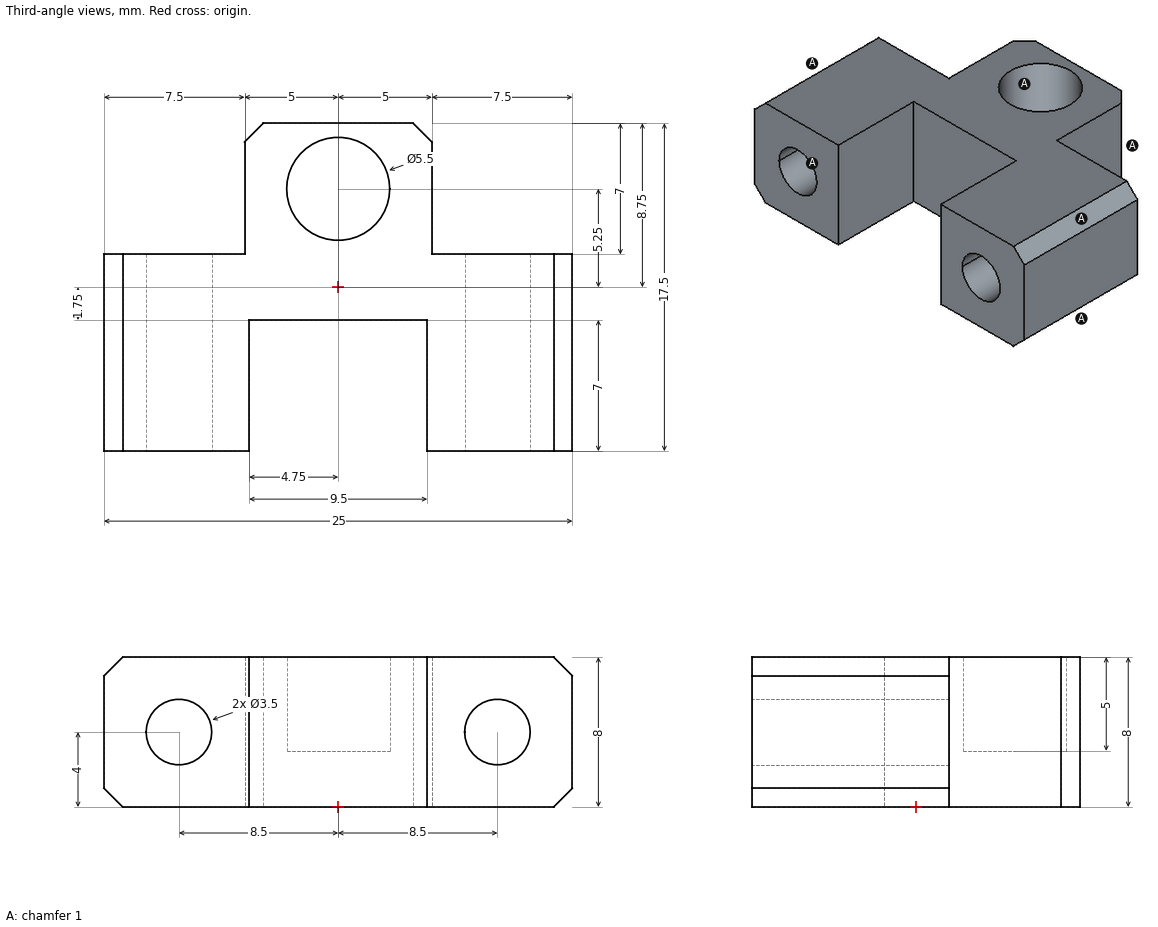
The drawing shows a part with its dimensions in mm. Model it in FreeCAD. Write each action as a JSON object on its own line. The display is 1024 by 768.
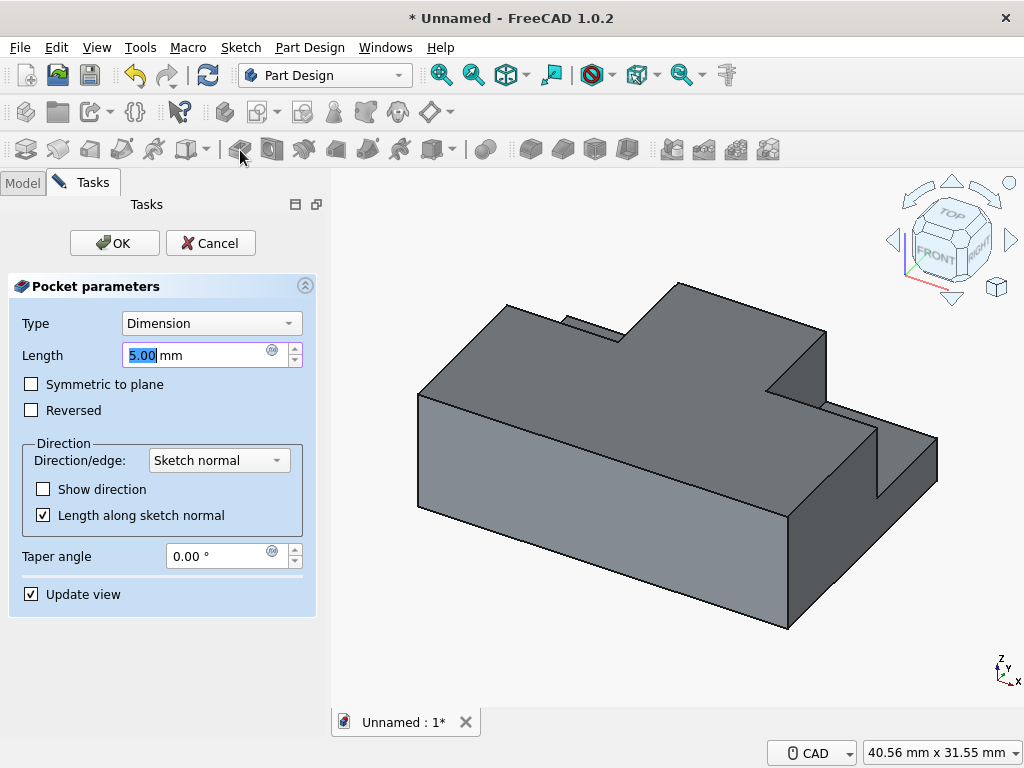
{"action": "type", "text": "8"}
{"action": "key", "text": "Tab"}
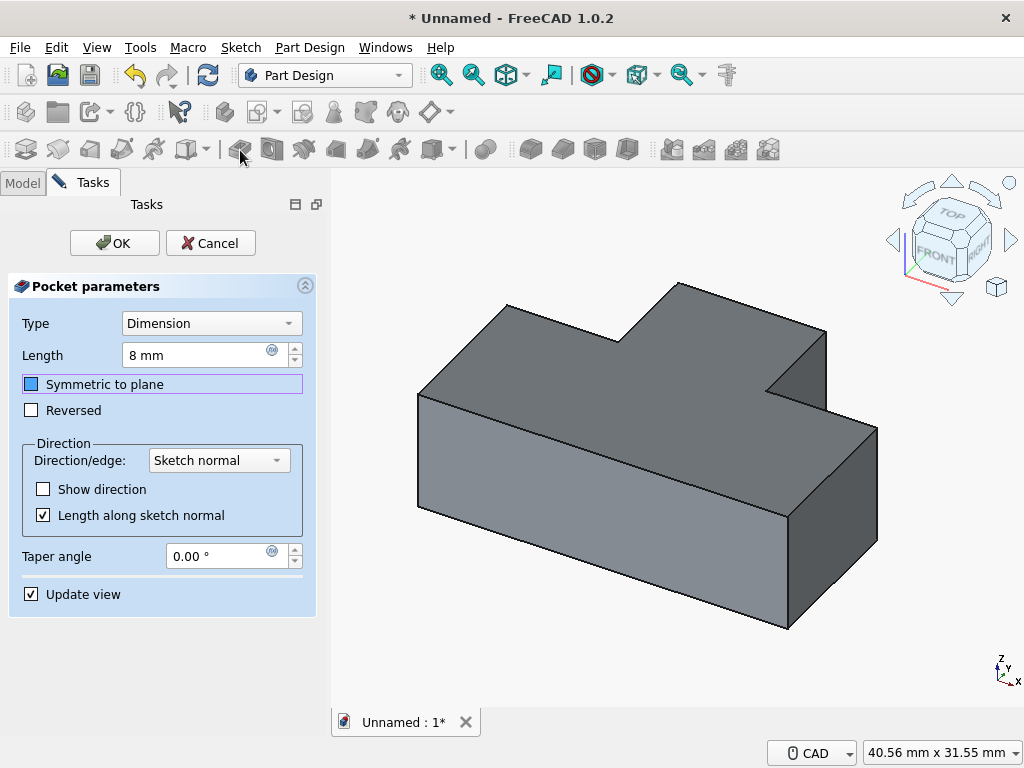
{"action": "left_click", "coordinate": [115, 243]}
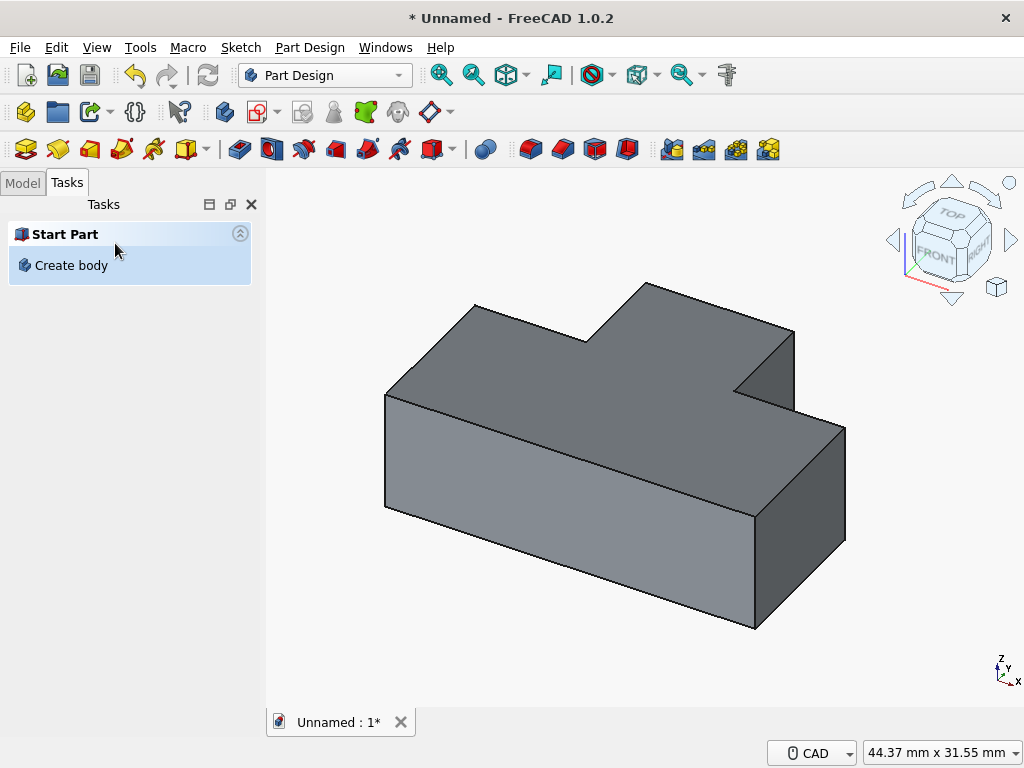
{"action": "left_click", "coordinate": [624, 402]}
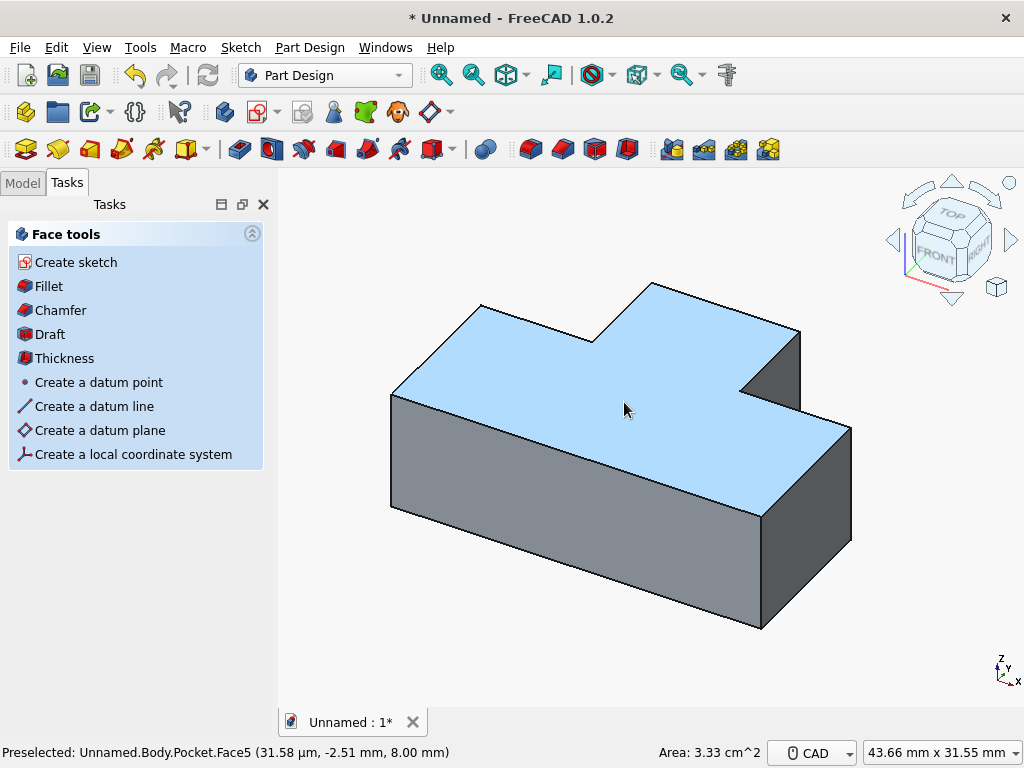
{"action": "left_click", "coordinate": [258, 112]}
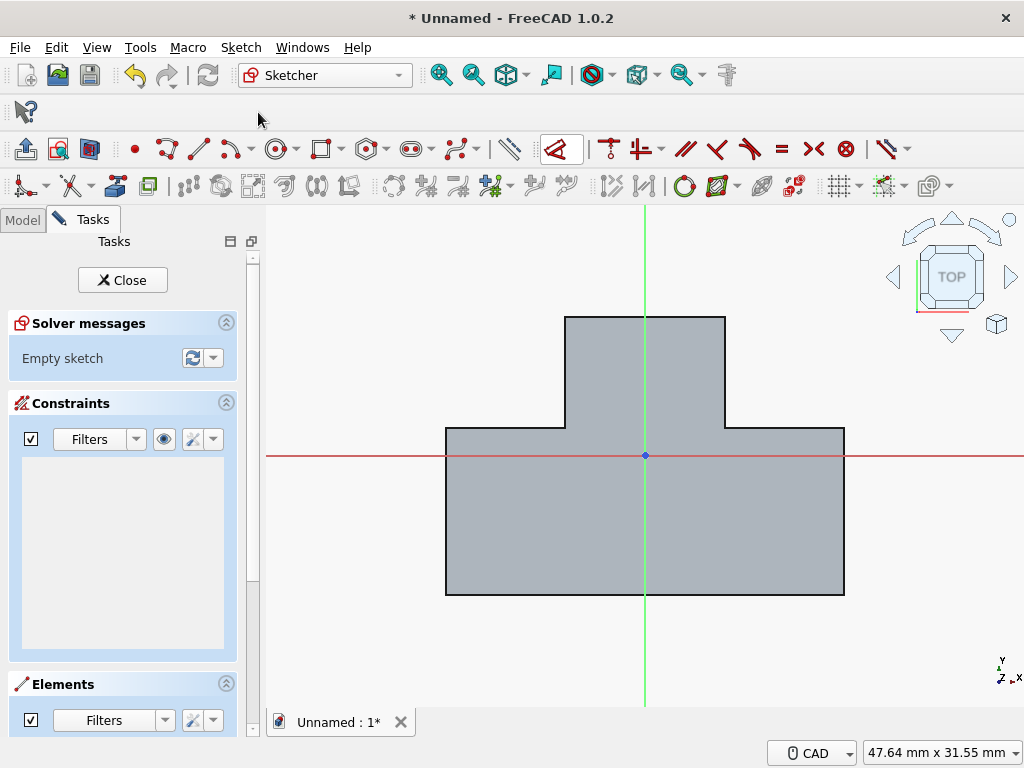
{"action": "scroll", "coordinate": [701, 582], "scroll_direction": "up", "scroll_amount": 4}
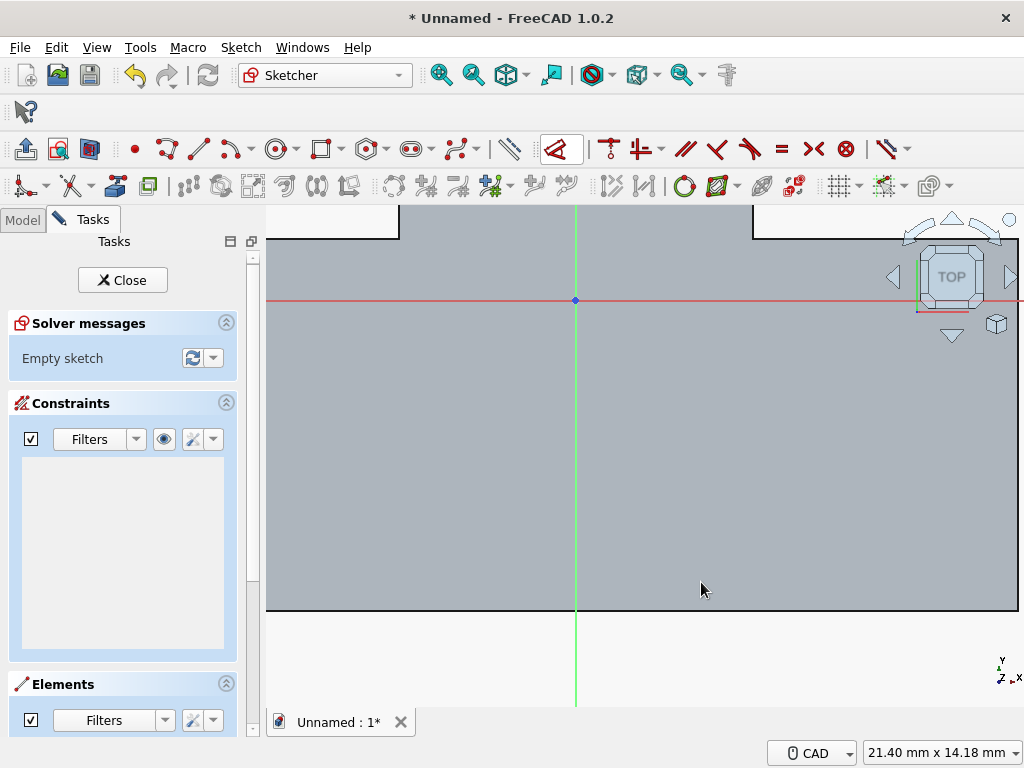
{"action": "key", "text": "g r"}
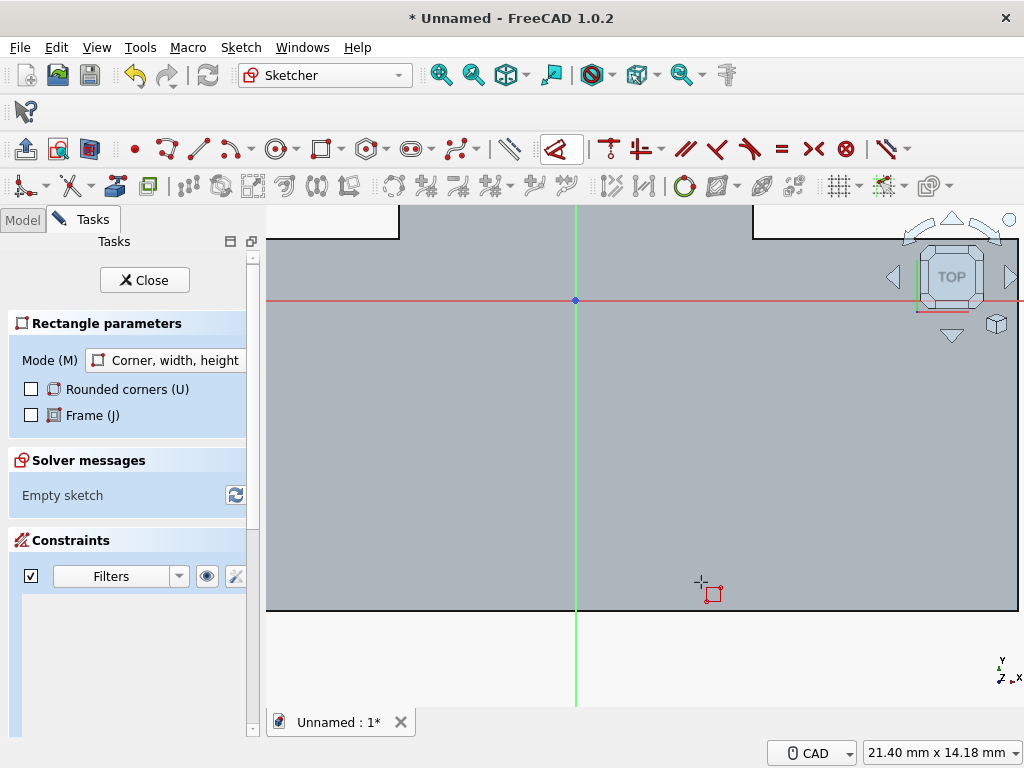
{"action": "left_click", "coordinate": [407, 363]}
{"action": "mouse_move", "coordinate": [744, 611]}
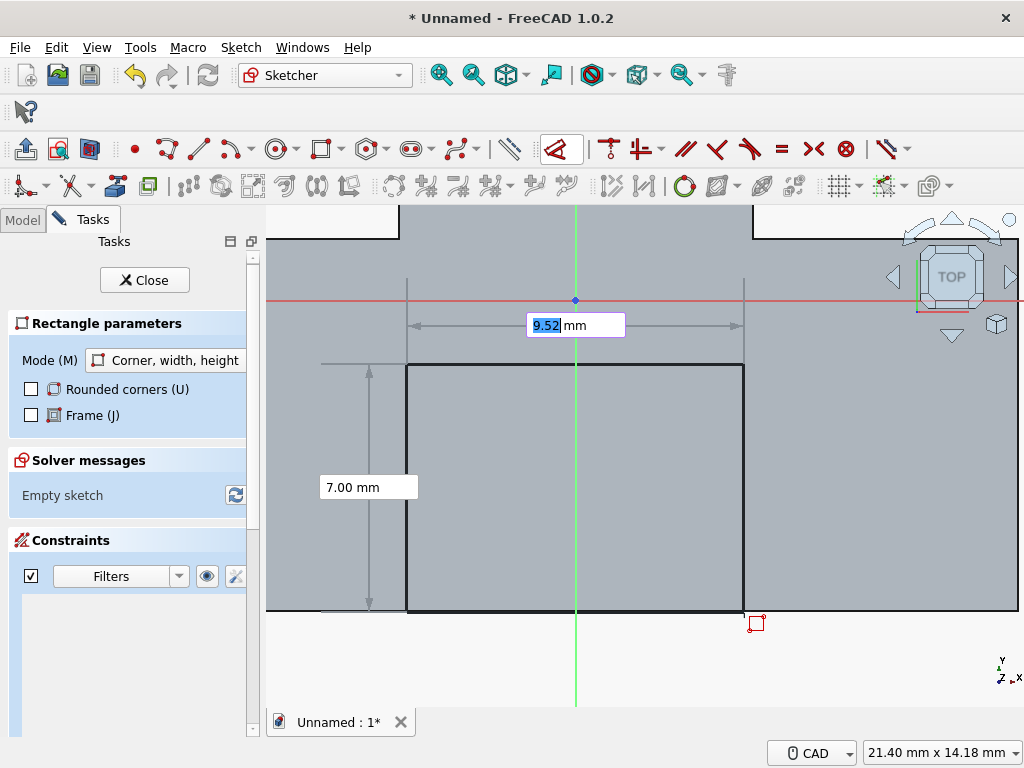
{"action": "type", "text": "9.5"}
{"action": "key", "text": "Tab"}
{"action": "type", "text": "7"}
{"action": "key", "text": "Return"}
{"action": "key", "text": "Escape"}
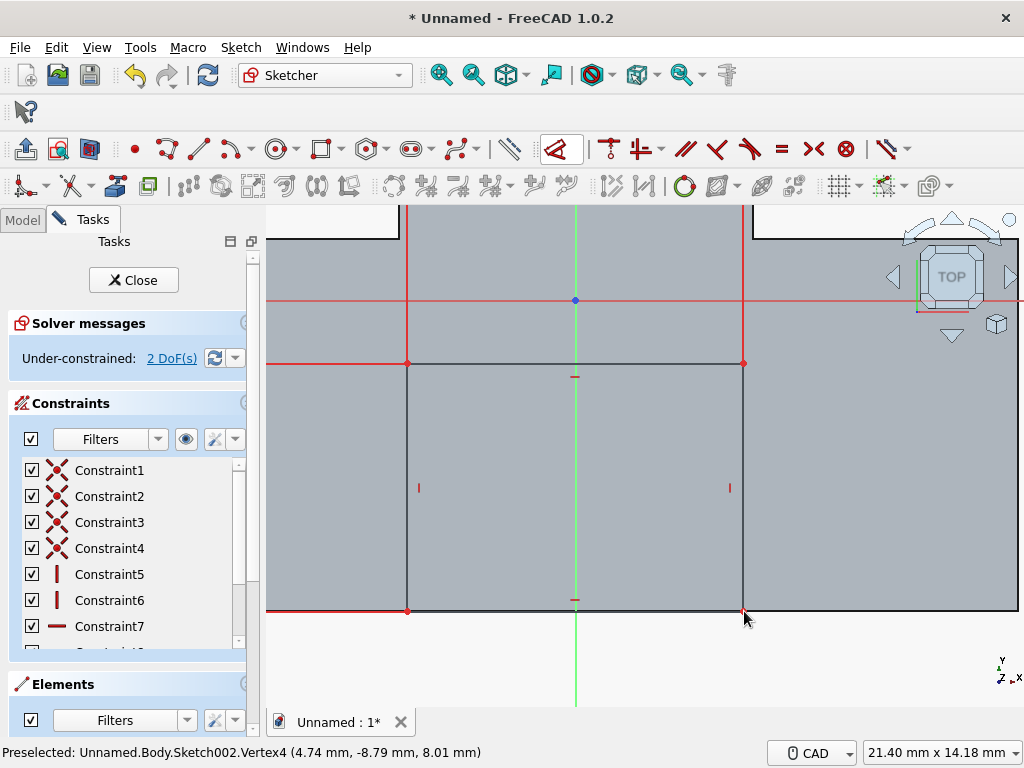
{"action": "left_click", "coordinate": [407, 364]}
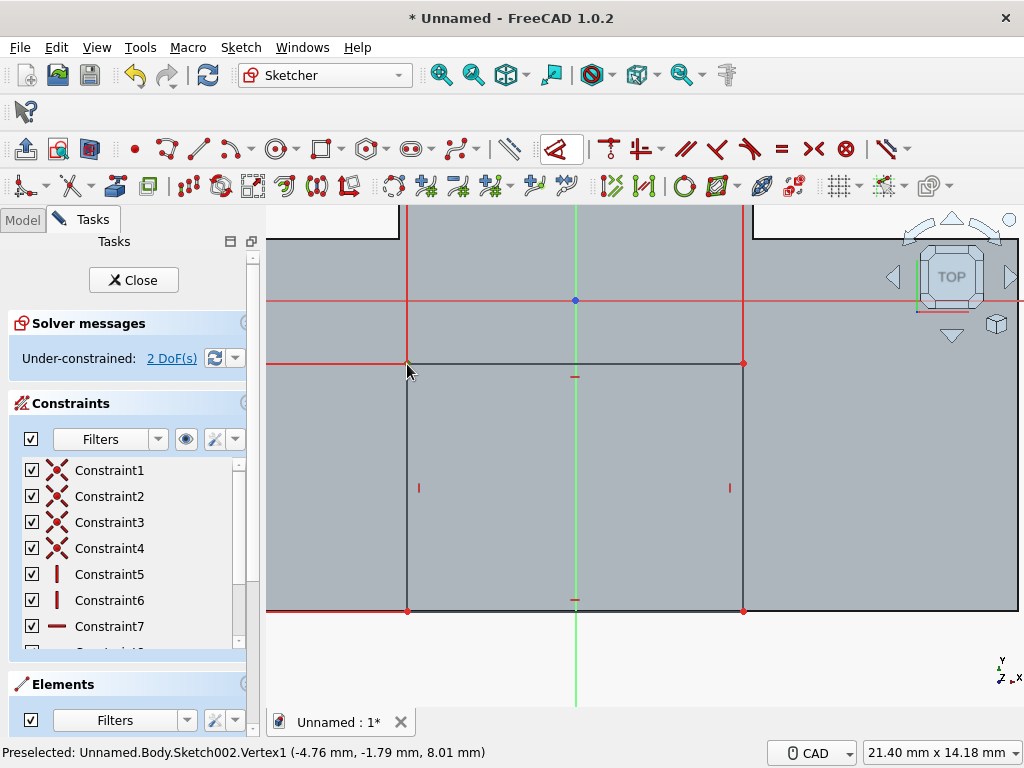
{"action": "key", "text": "l"}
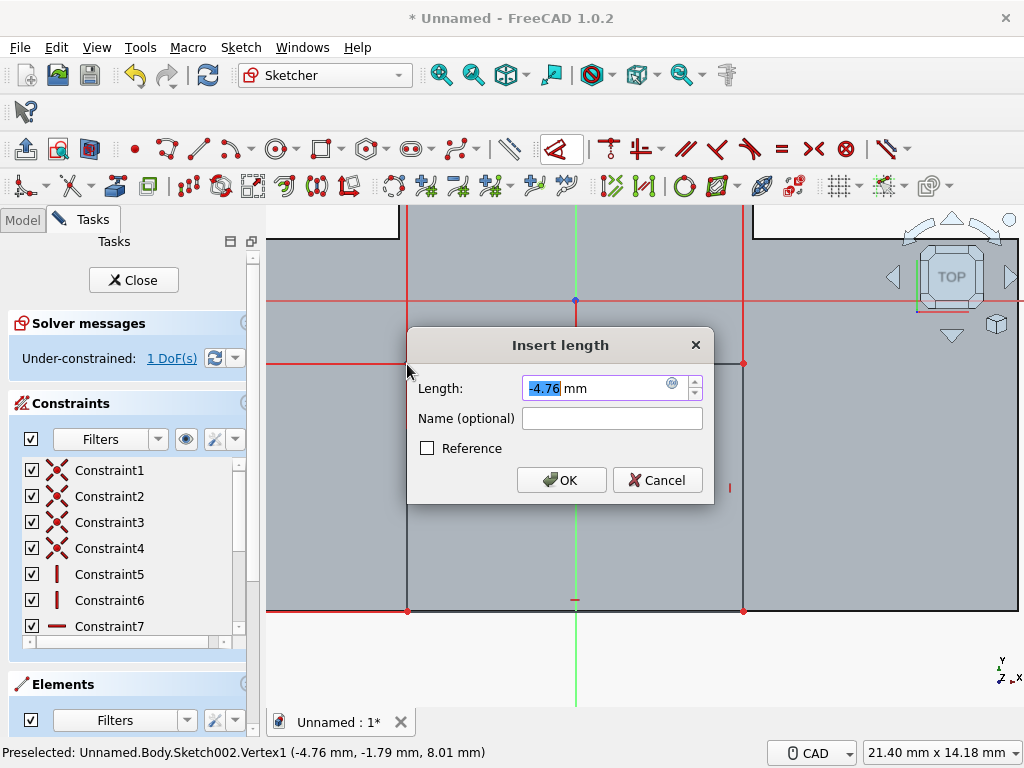
{"action": "type", "text": "-4.75"}
{"action": "key", "text": "Return"}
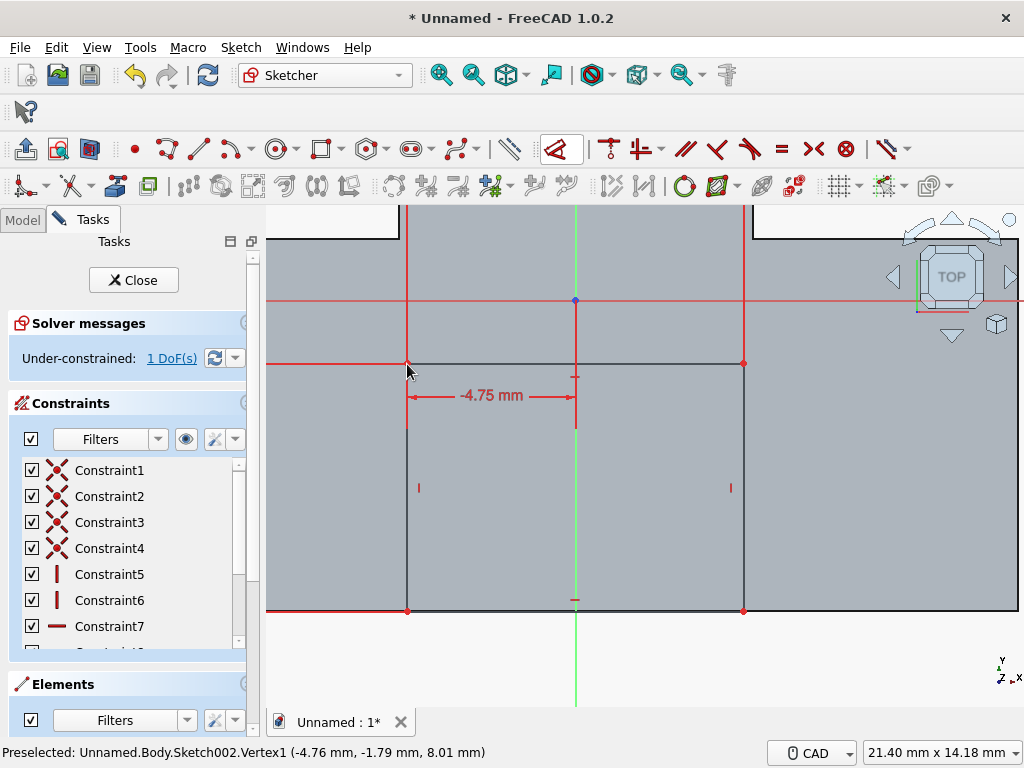
{"action": "left_click", "coordinate": [407, 364]}